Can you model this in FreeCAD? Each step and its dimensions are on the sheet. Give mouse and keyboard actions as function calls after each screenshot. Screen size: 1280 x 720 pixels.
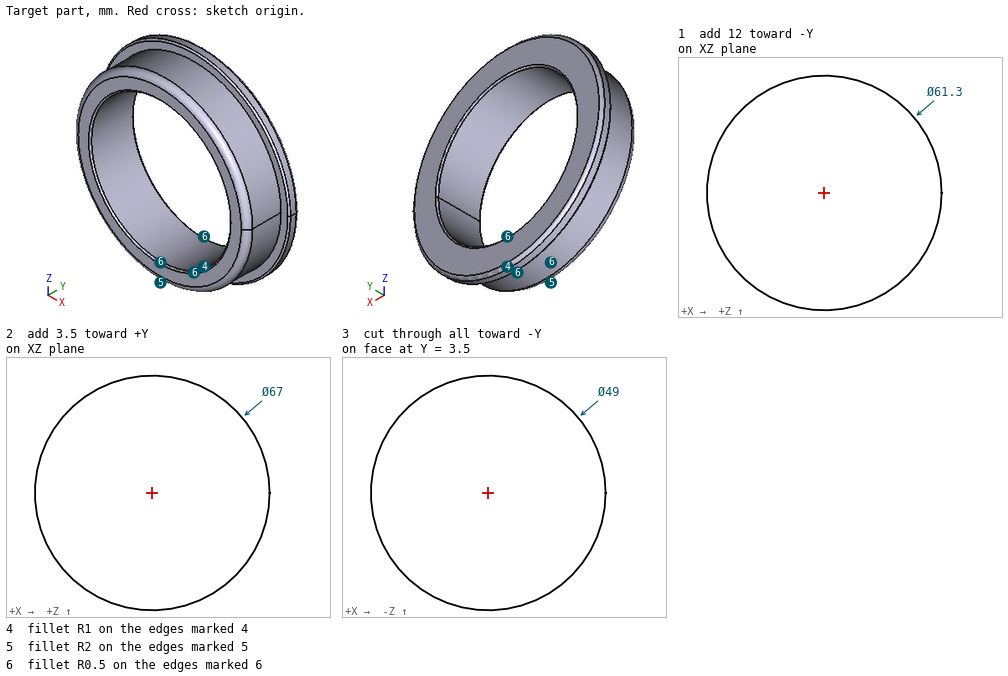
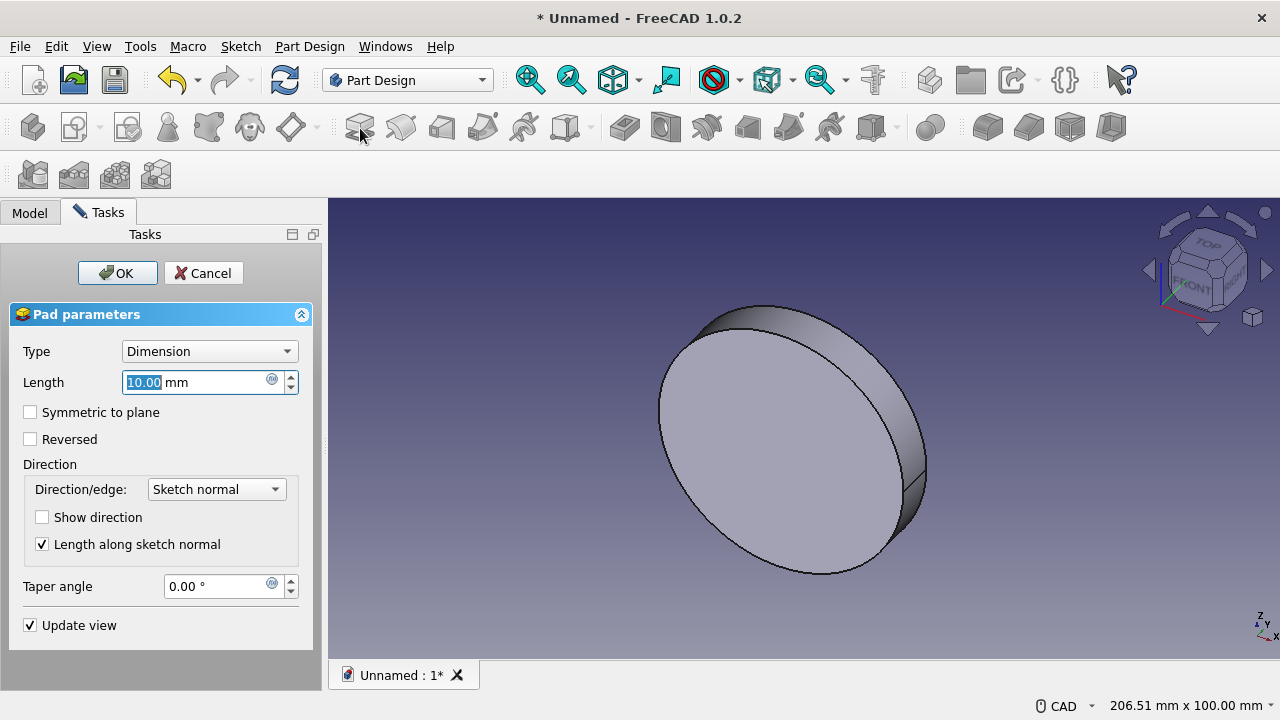
text(12)
key(Tab)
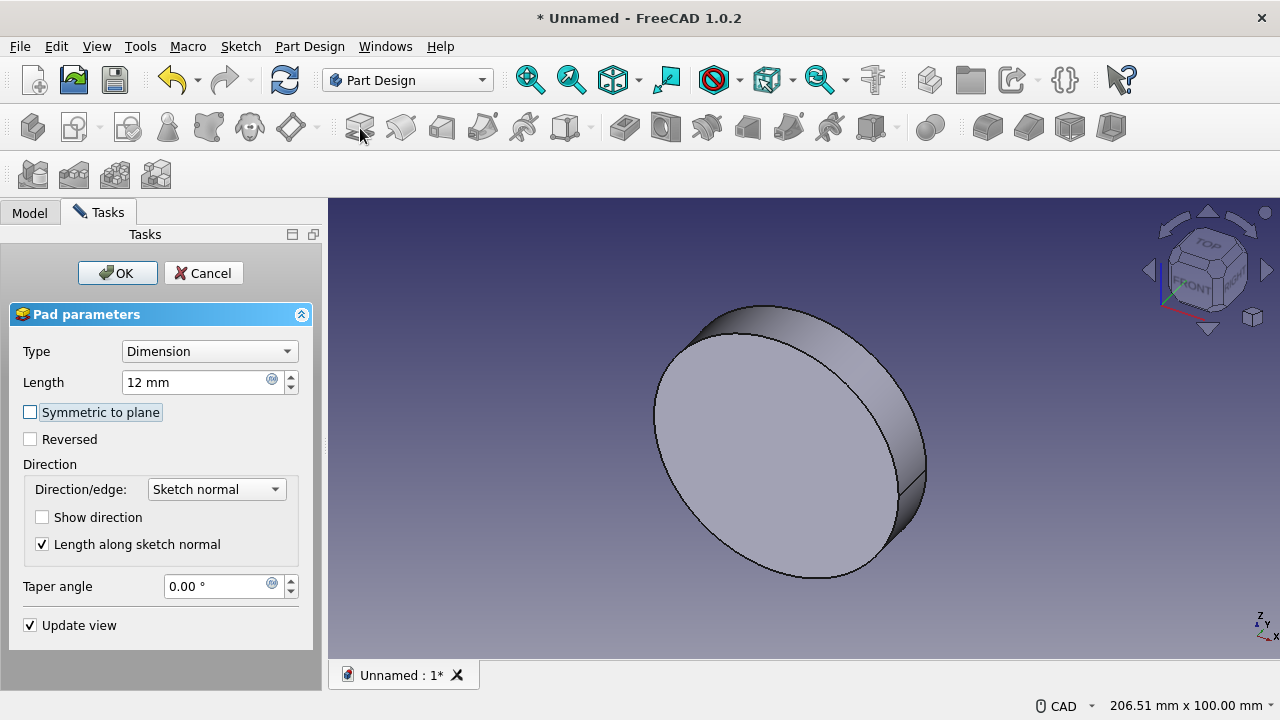
click(118, 273)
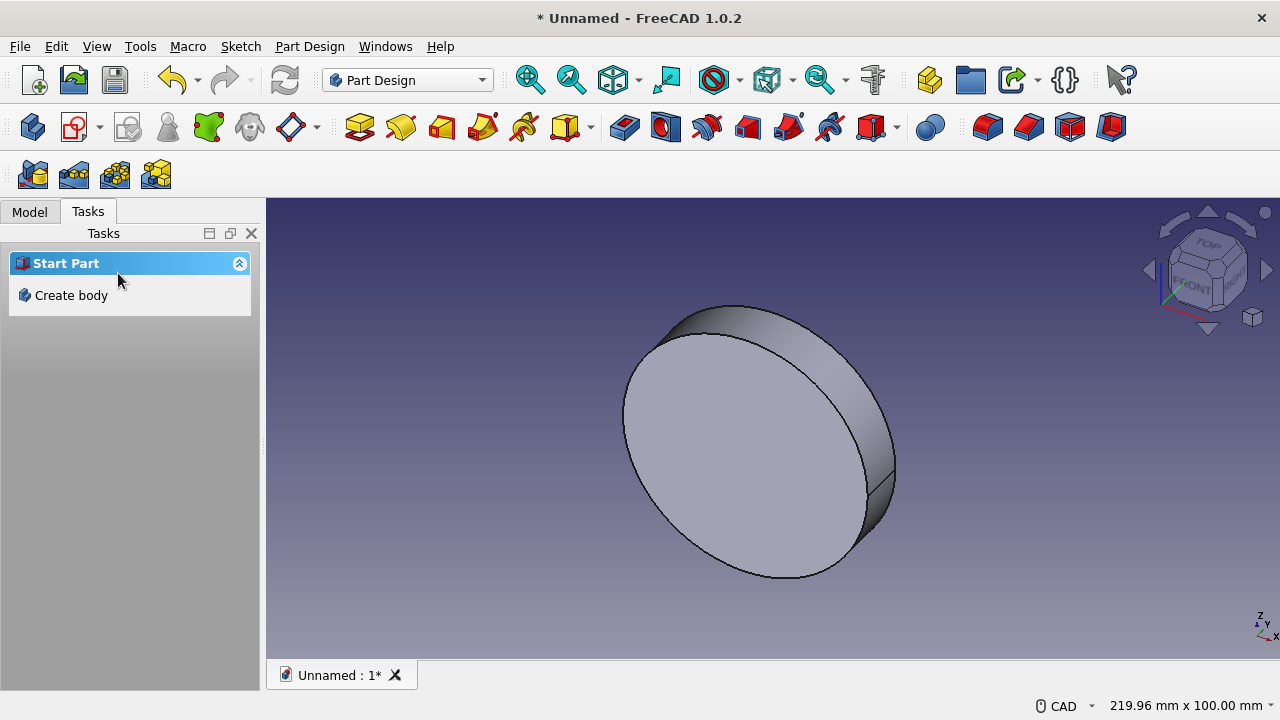
click(74, 128)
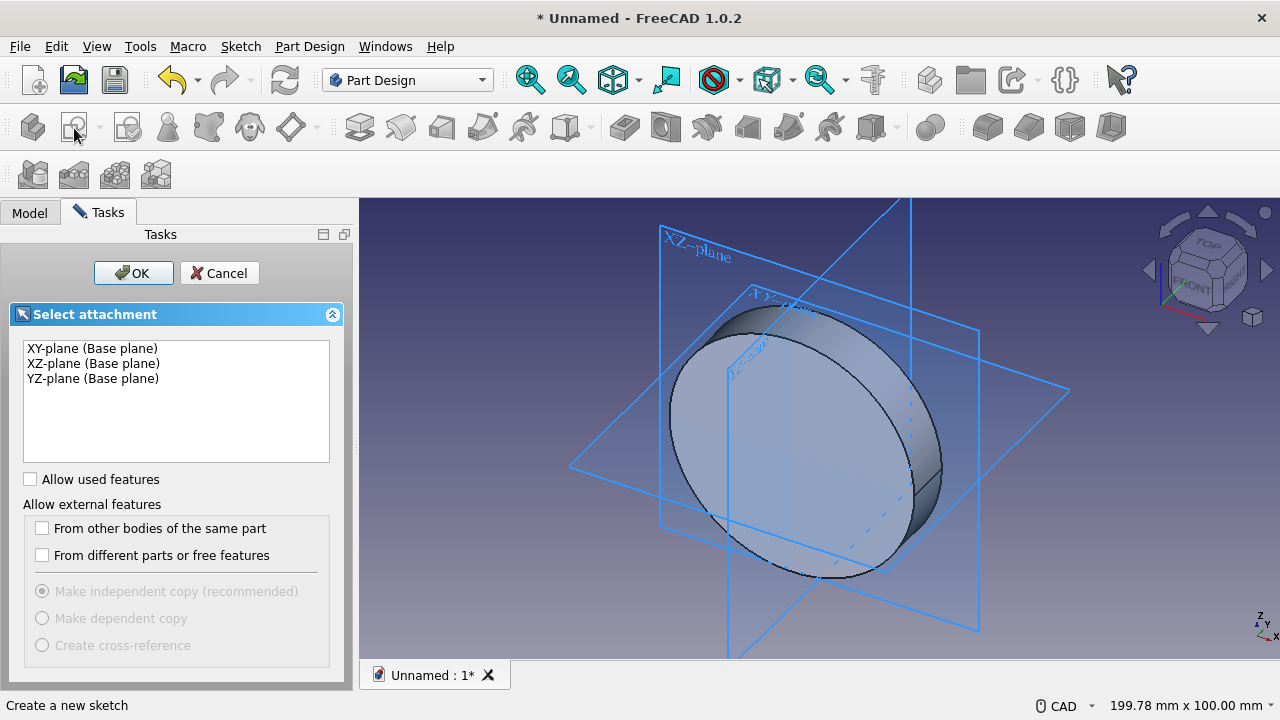
click(84, 364)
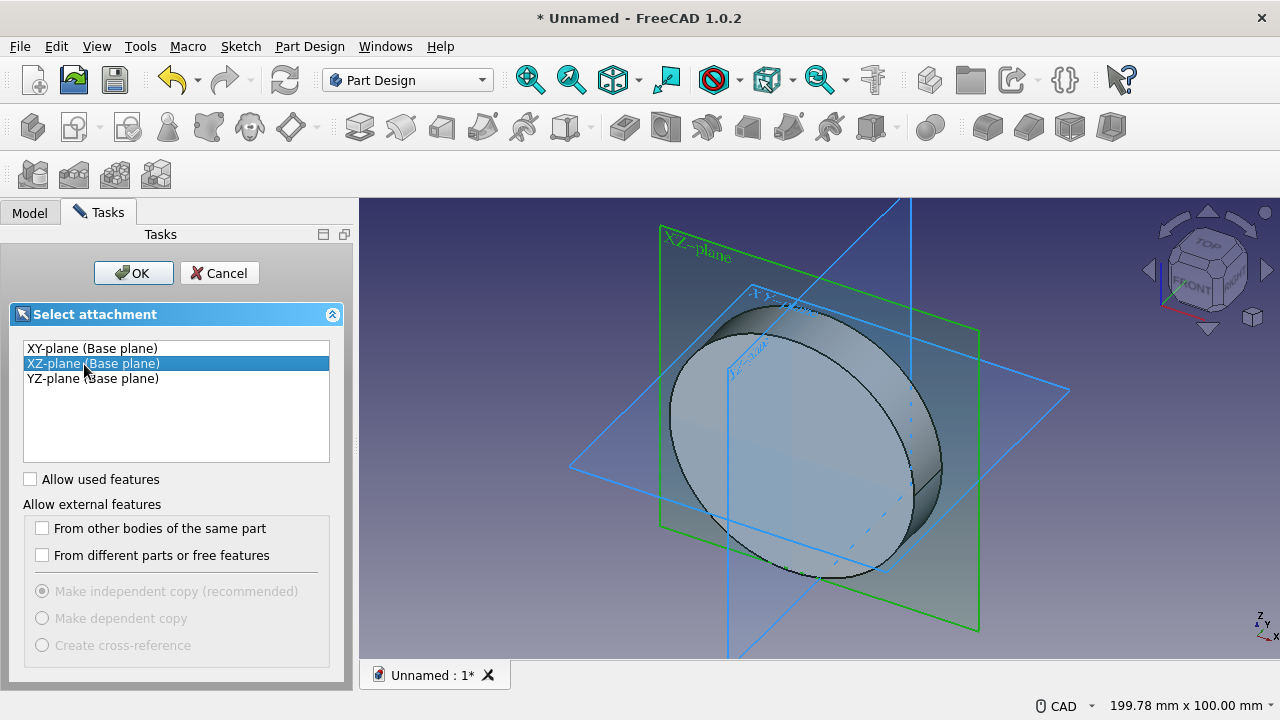
click(134, 273)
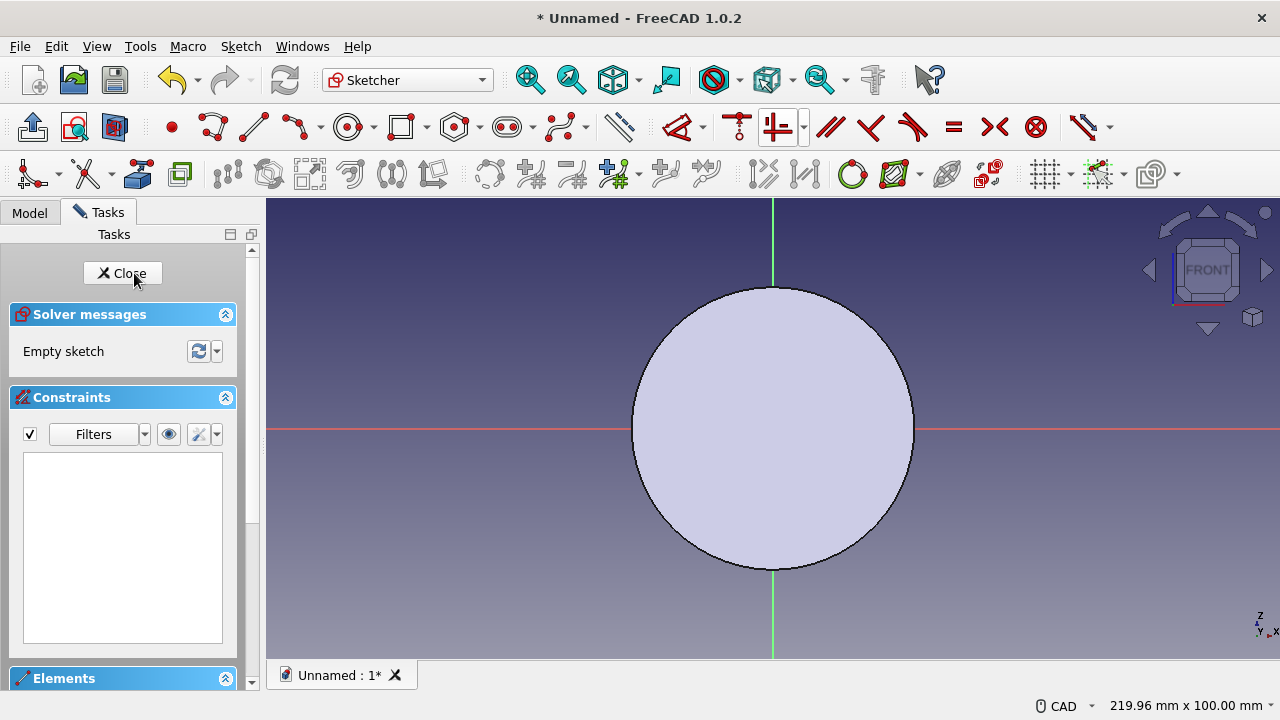
click(115, 128)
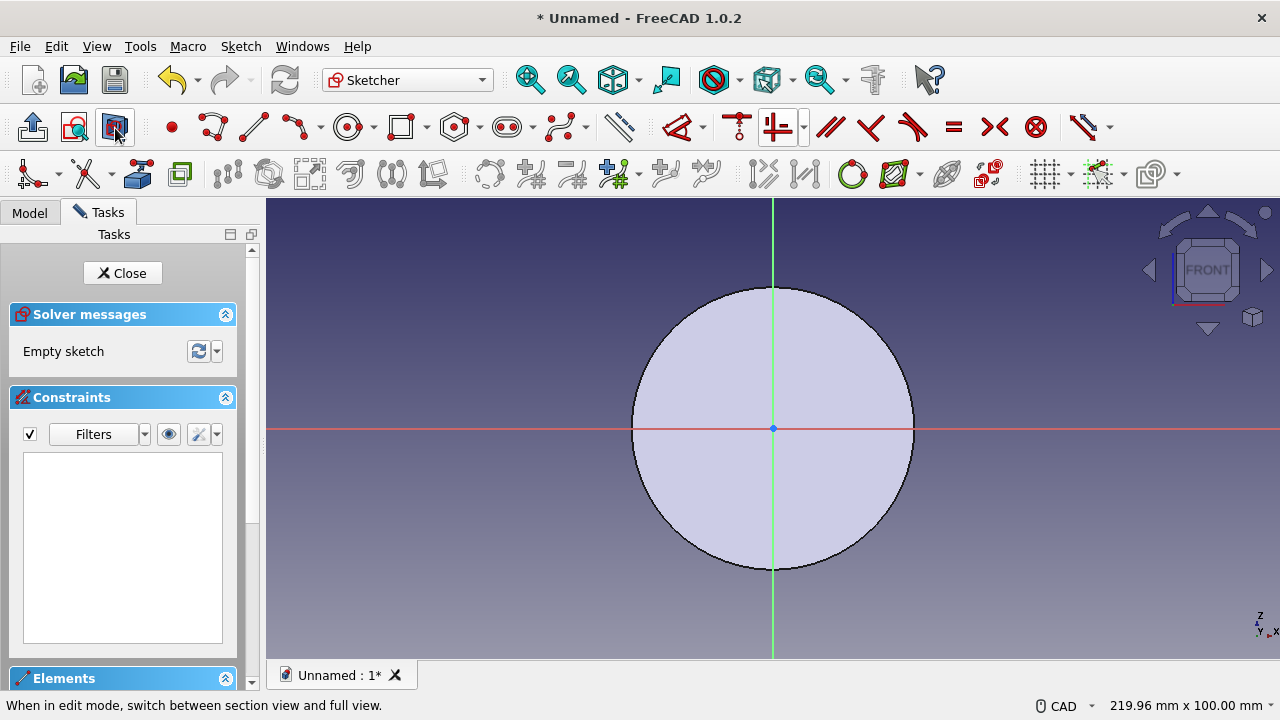
click(348, 128)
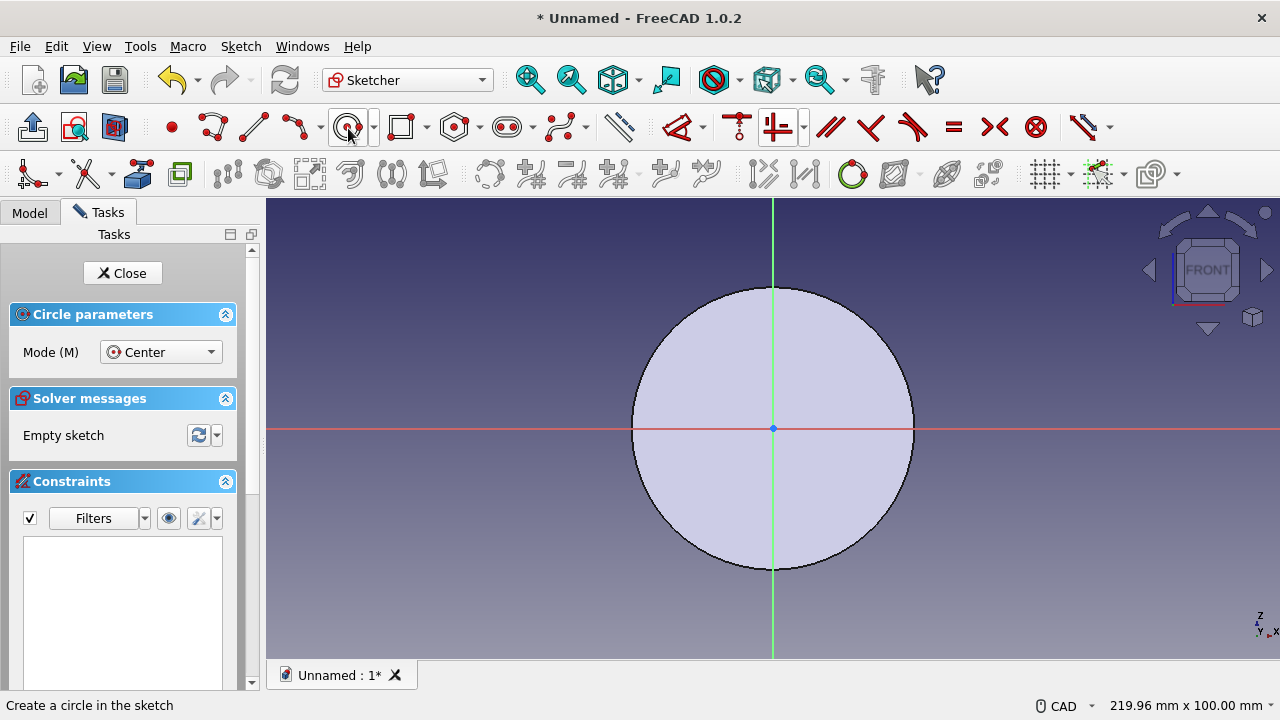
click(773, 428)
click(882, 319)
key(Escape)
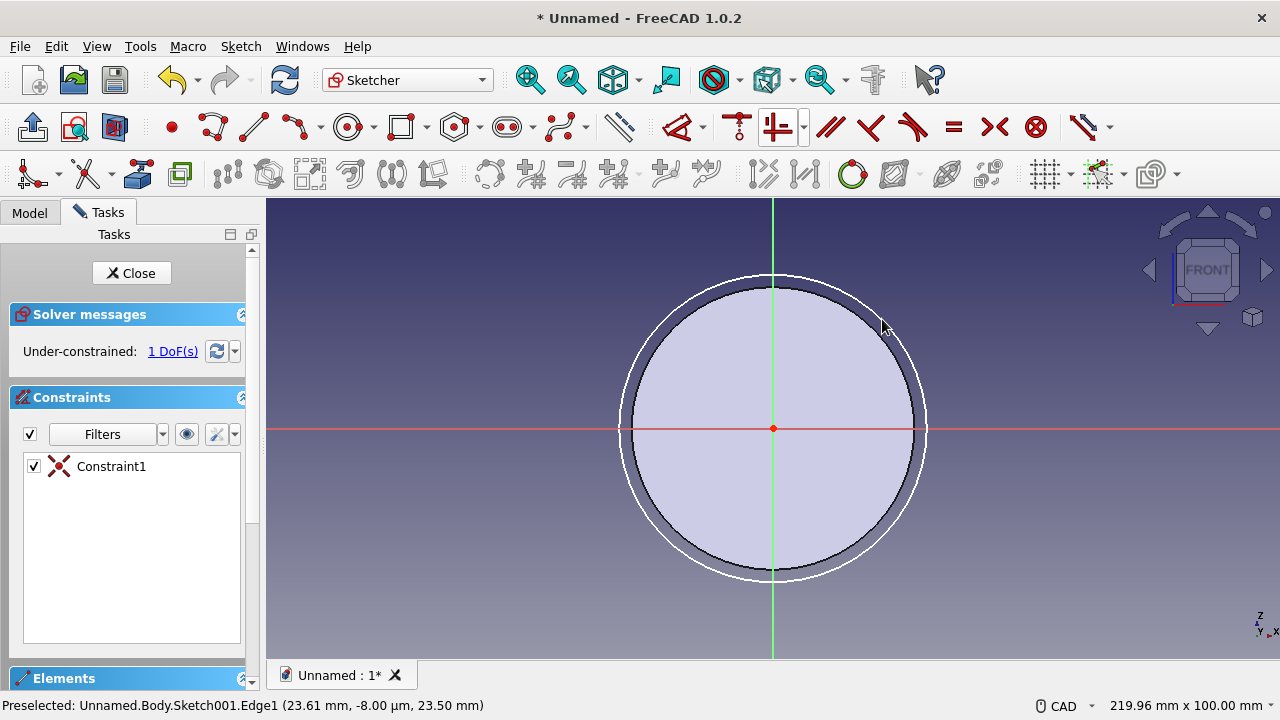
click(676, 128)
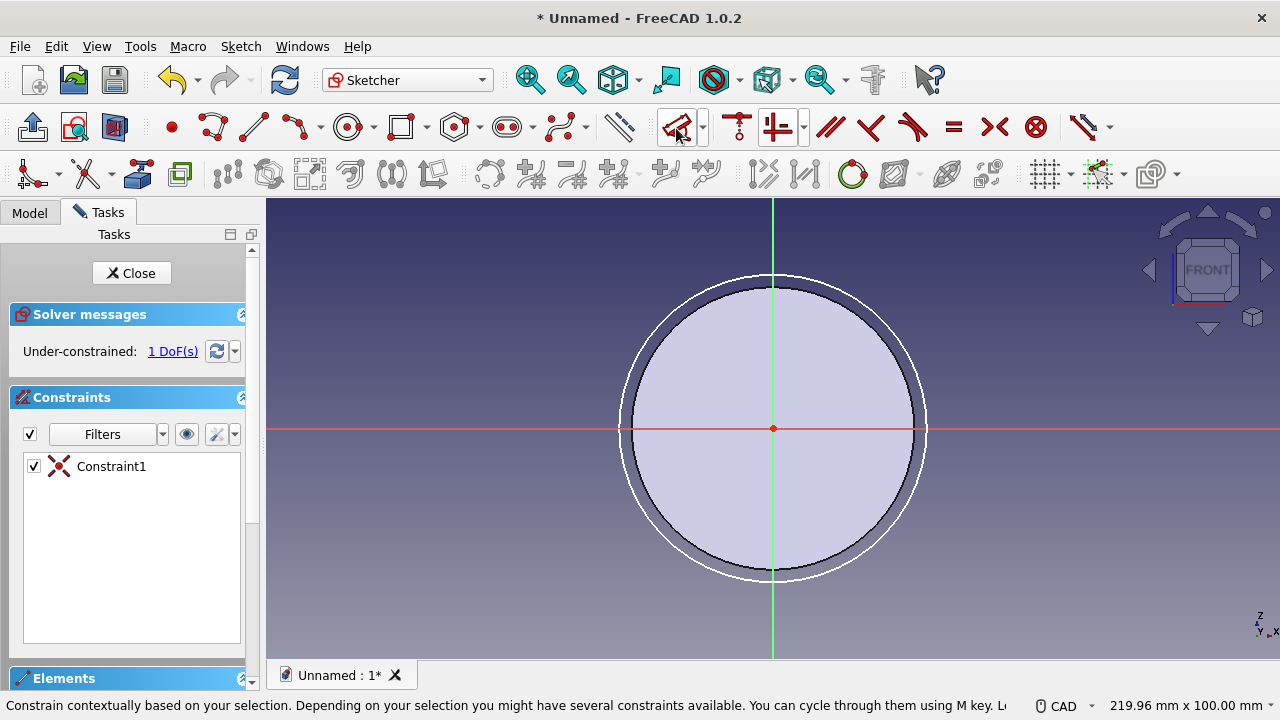
click(881, 319)
click(903, 296)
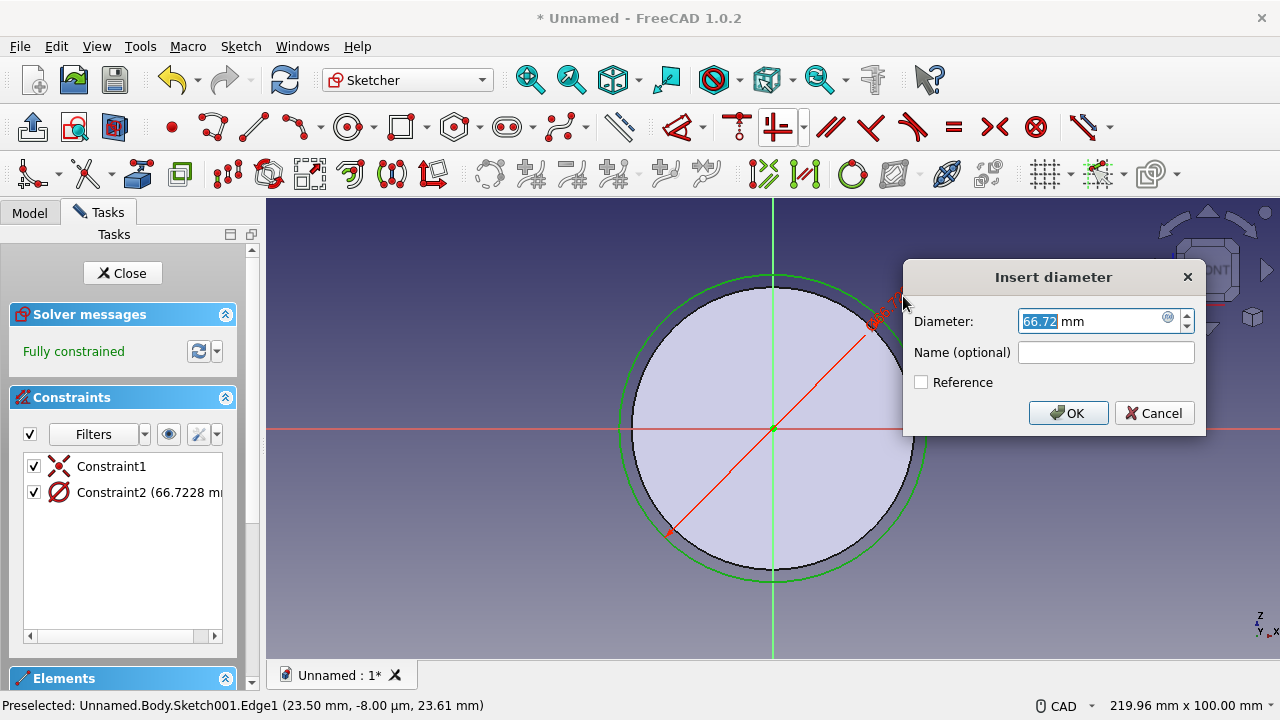
text(67)
key(Return)
key(Escape)